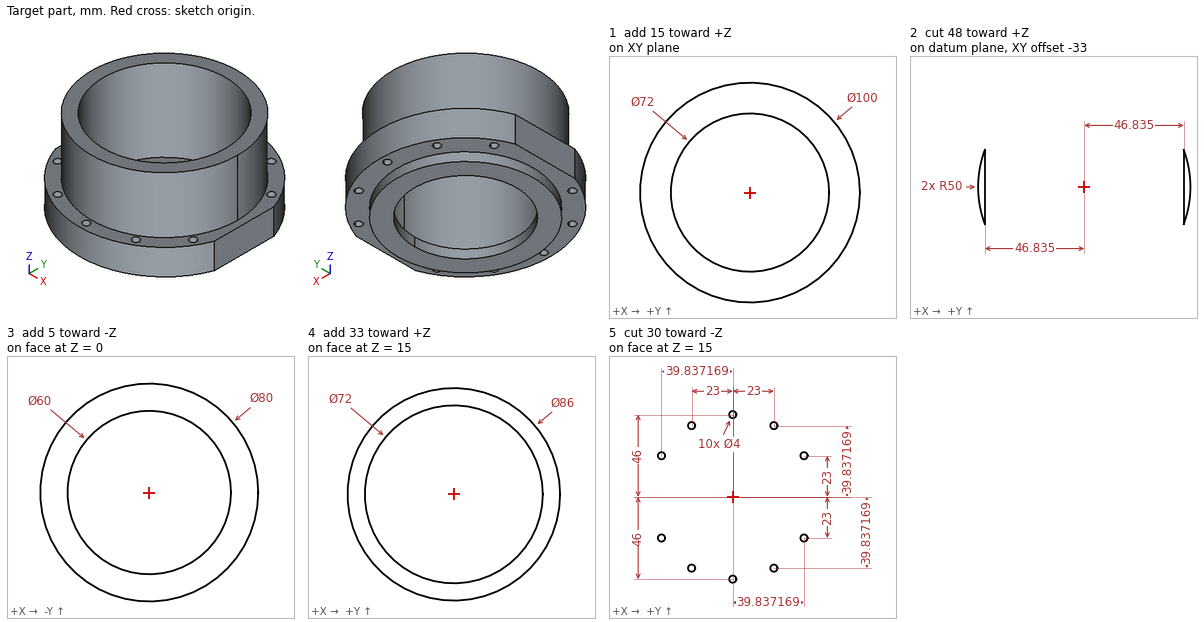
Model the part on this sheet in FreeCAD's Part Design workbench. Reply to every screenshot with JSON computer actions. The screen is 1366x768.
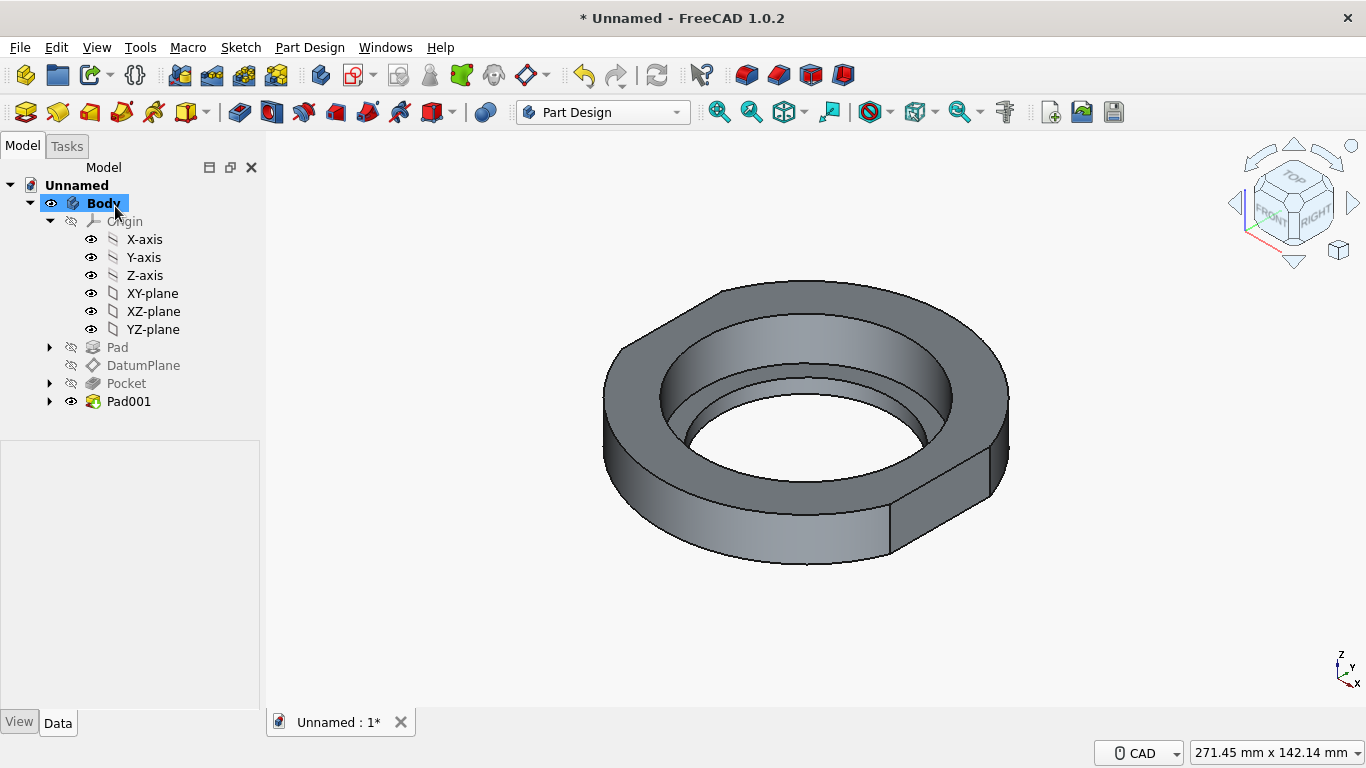
{"action": "left_click", "coordinate": [929, 326]}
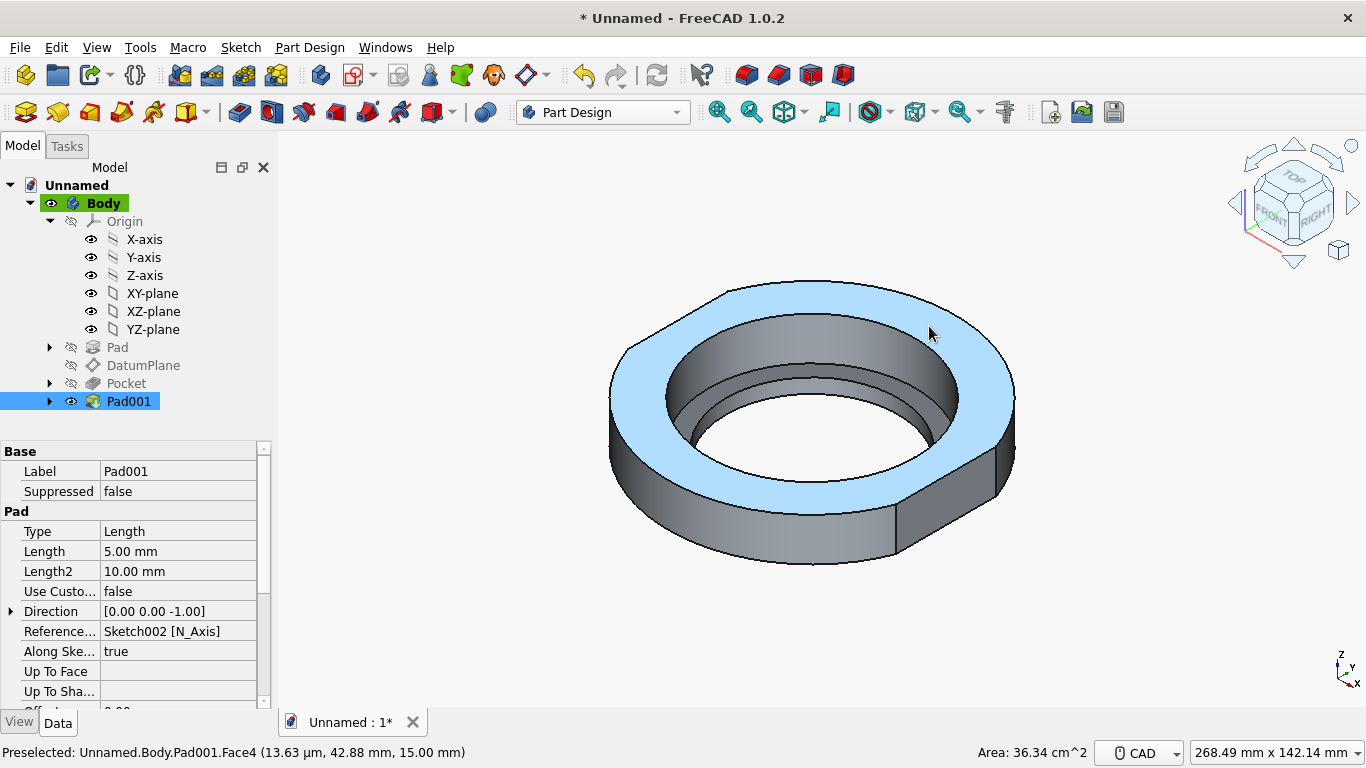
{"action": "left_click", "coordinate": [354, 76]}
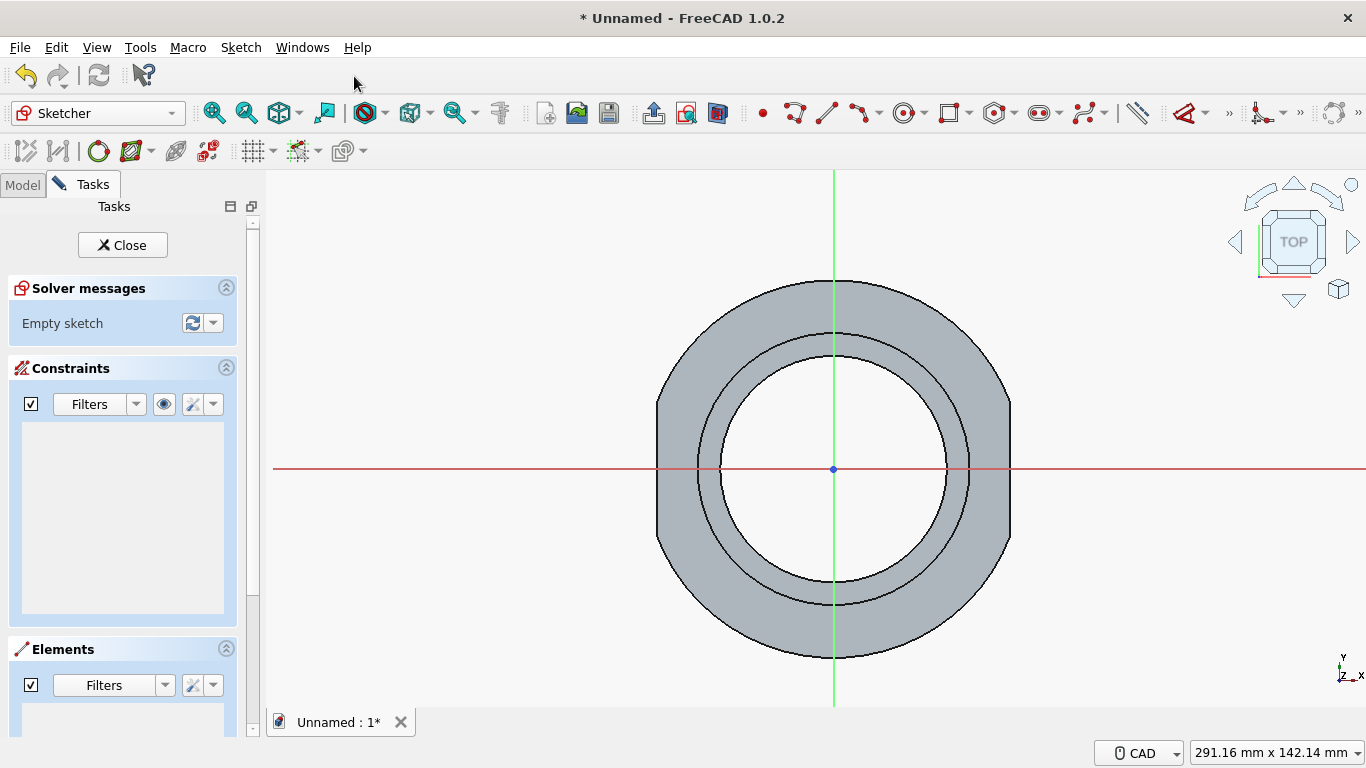
{"action": "left_click", "coordinate": [904, 114]}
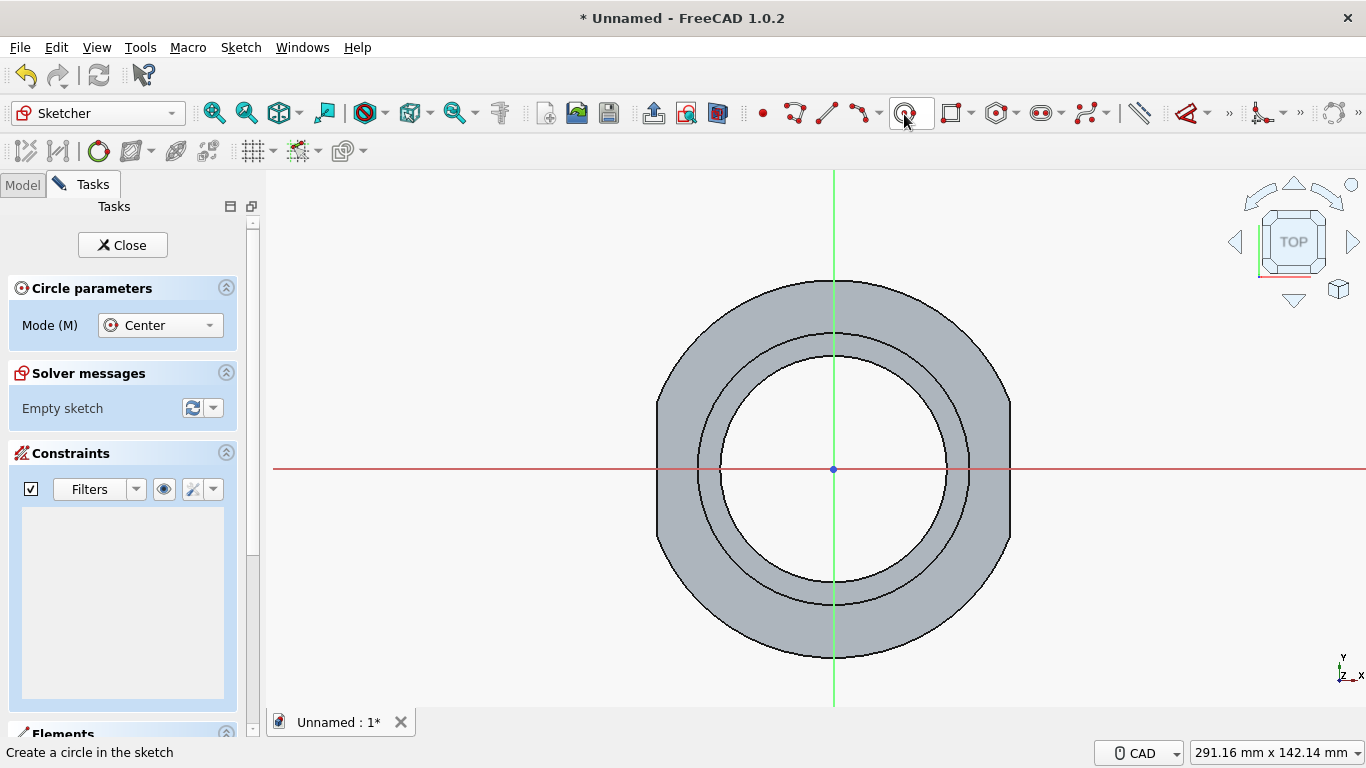
{"action": "left_click", "coordinate": [834, 469]}
{"action": "mouse_move", "coordinate": [948, 354]}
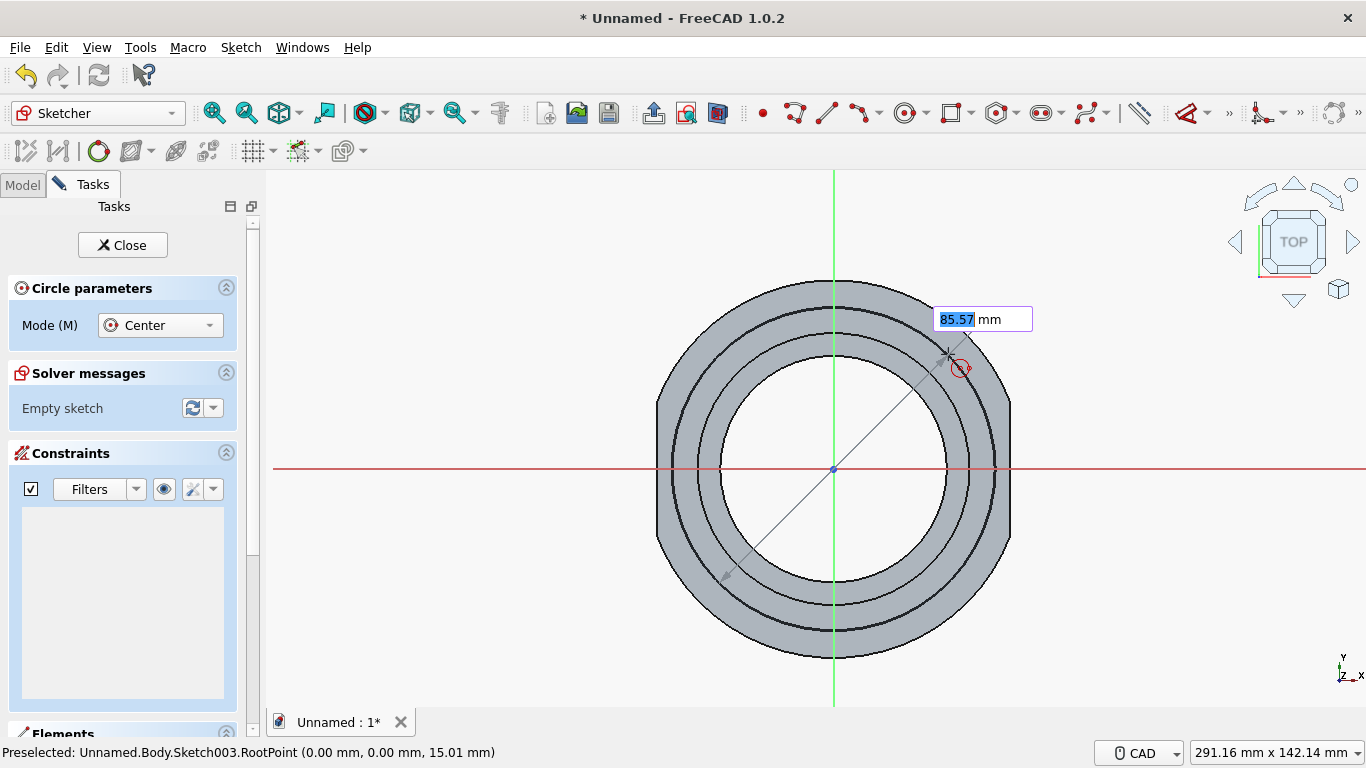
{"action": "type", "text": "86"}
{"action": "key", "text": "Return"}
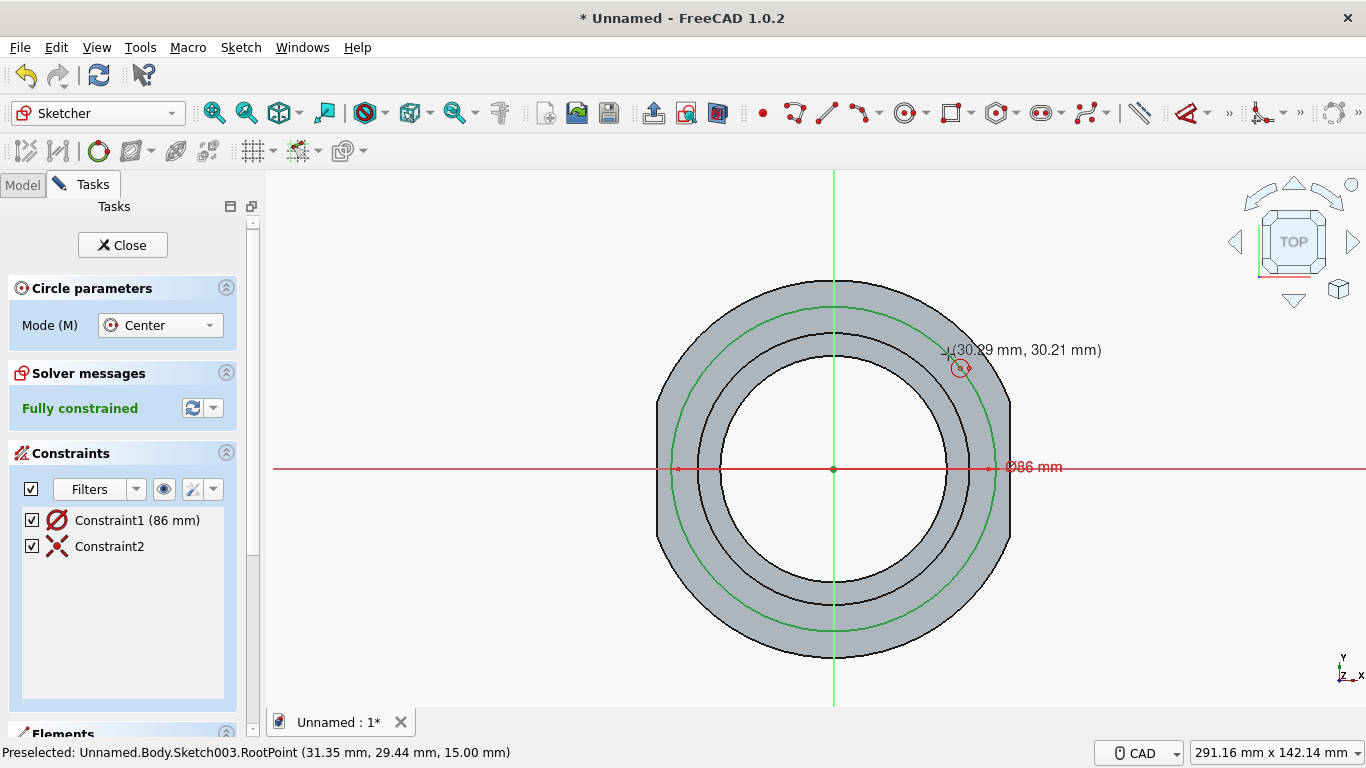
{"action": "left_click", "coordinate": [834, 469]}
{"action": "mouse_move", "coordinate": [930, 373]}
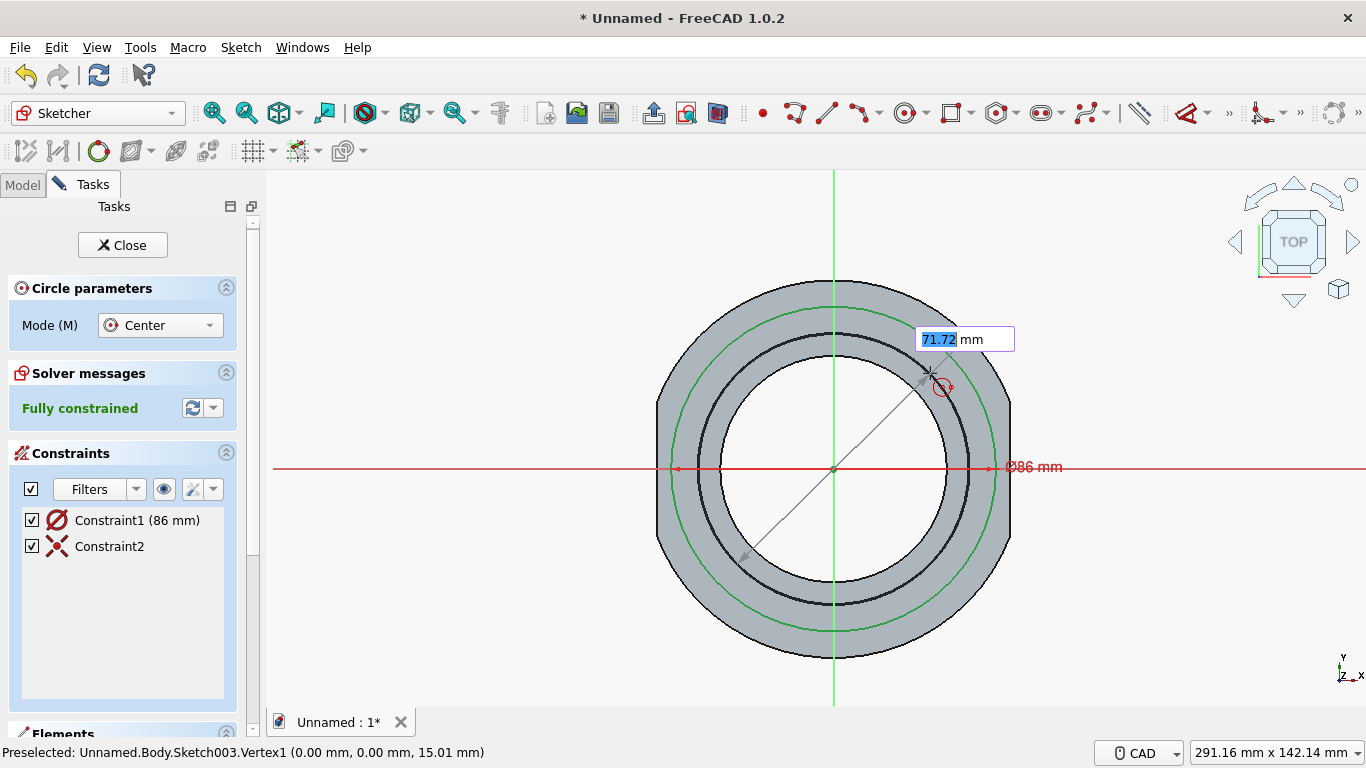
{"action": "type", "text": "72"}
{"action": "key", "text": "Return"}
{"action": "key", "text": "Escape"}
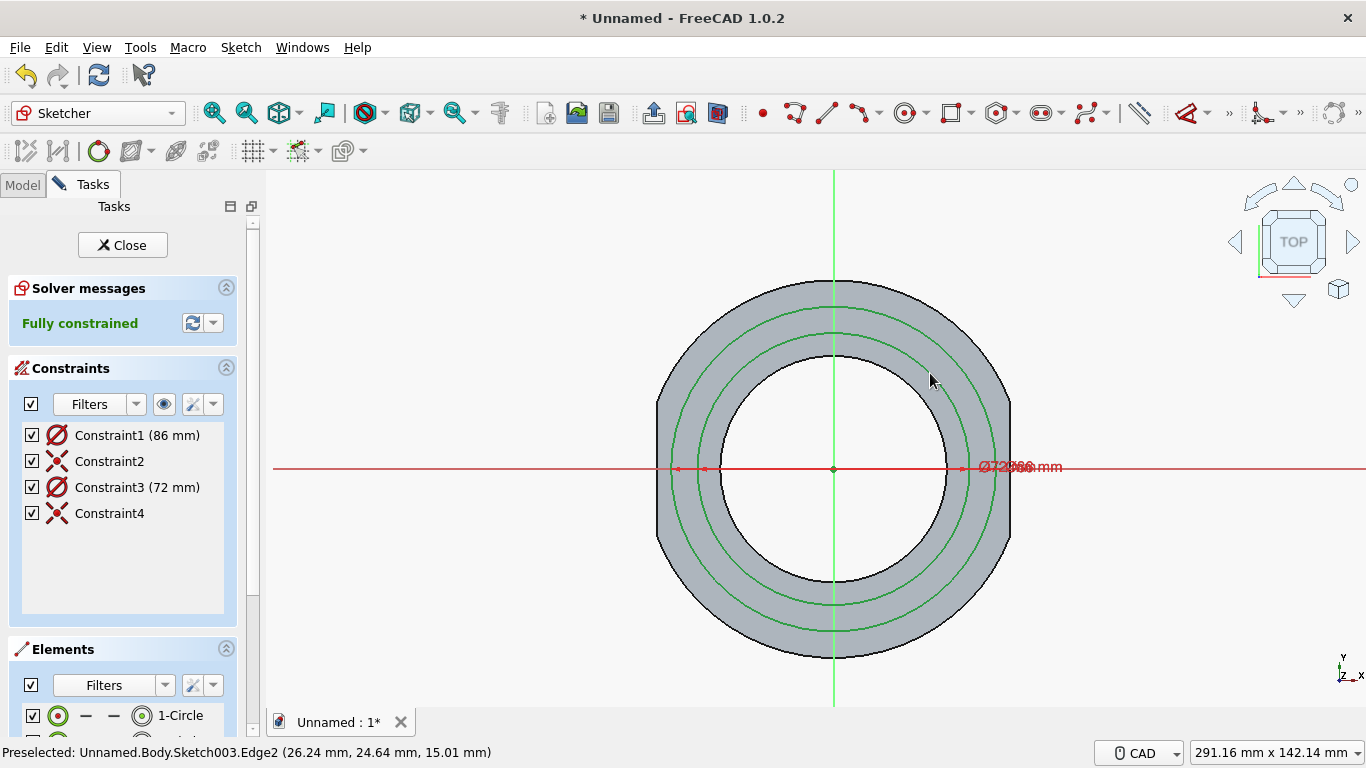
{"action": "left_click", "coordinate": [123, 245]}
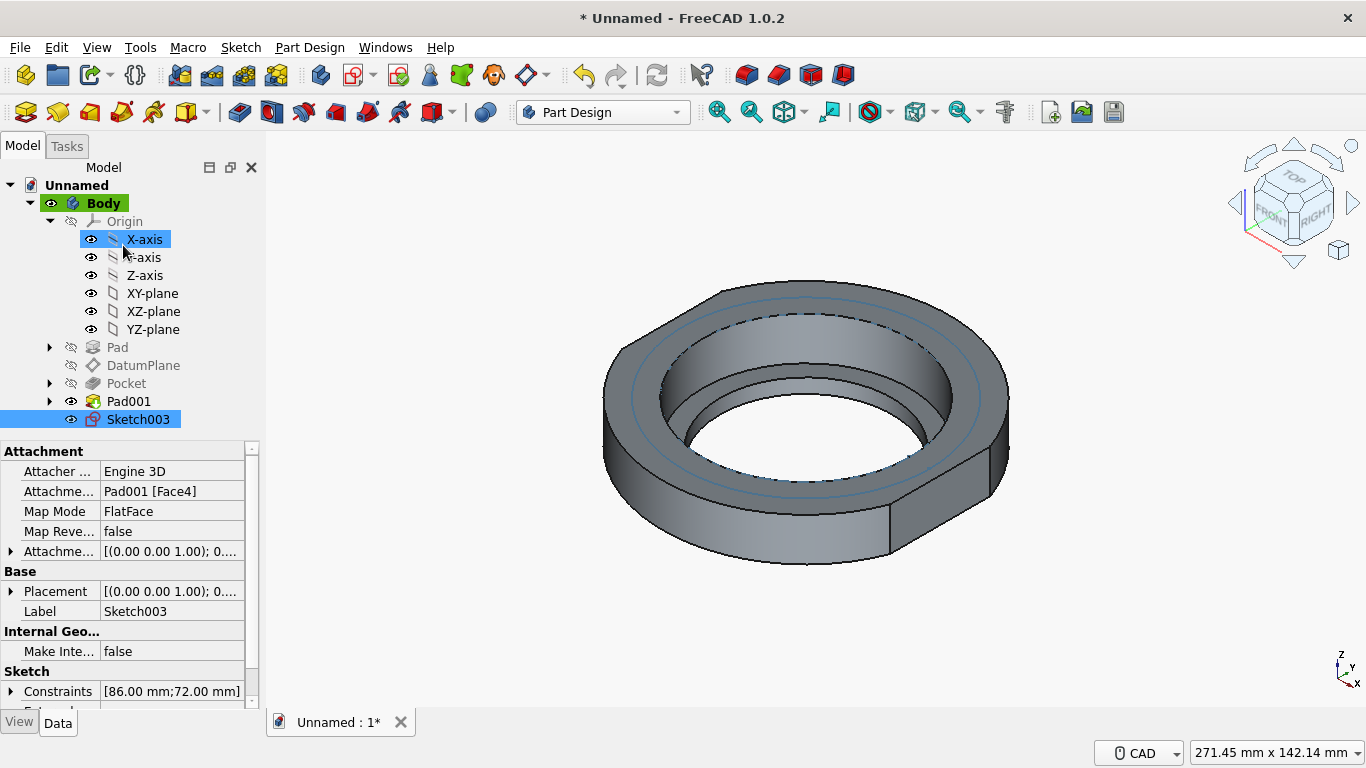
{"action": "left_click", "coordinate": [26, 112]}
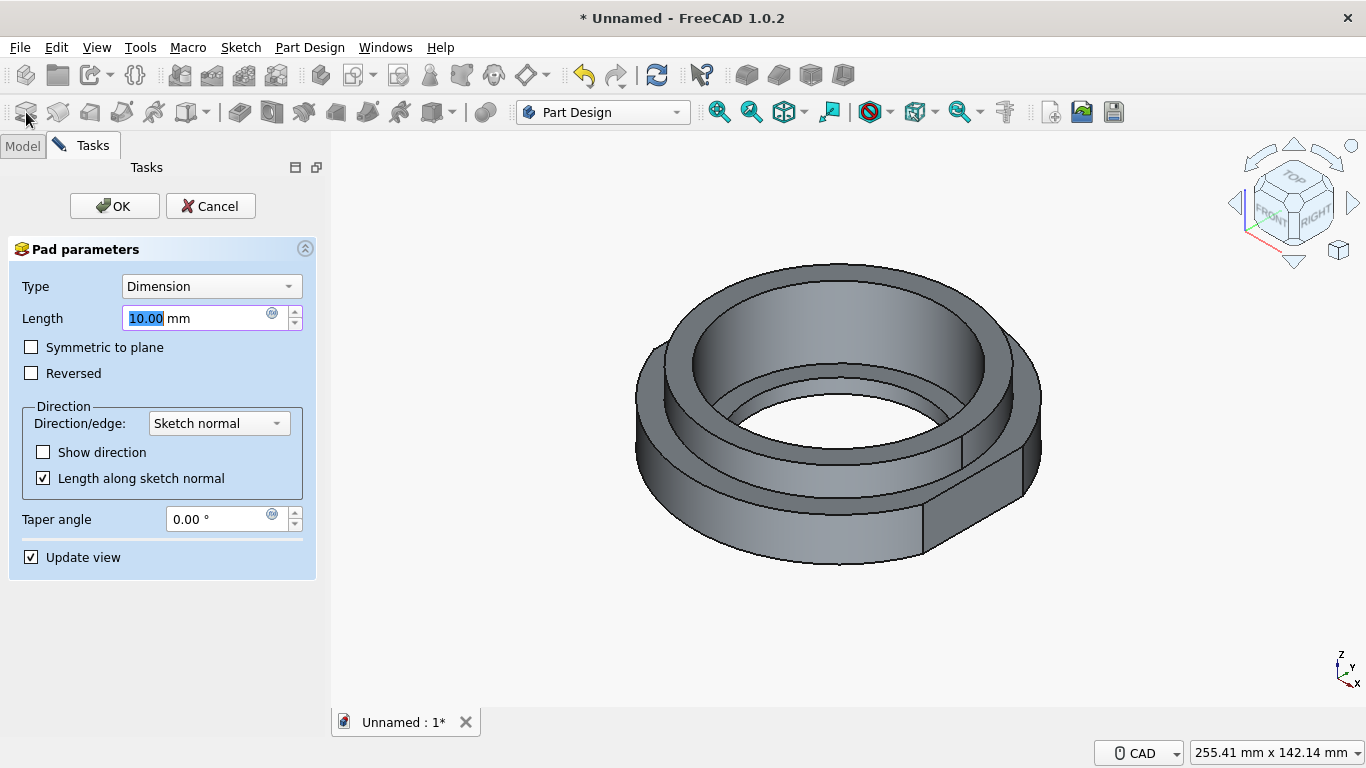
{"action": "type", "text": "33"}
{"action": "key", "text": "Tab"}